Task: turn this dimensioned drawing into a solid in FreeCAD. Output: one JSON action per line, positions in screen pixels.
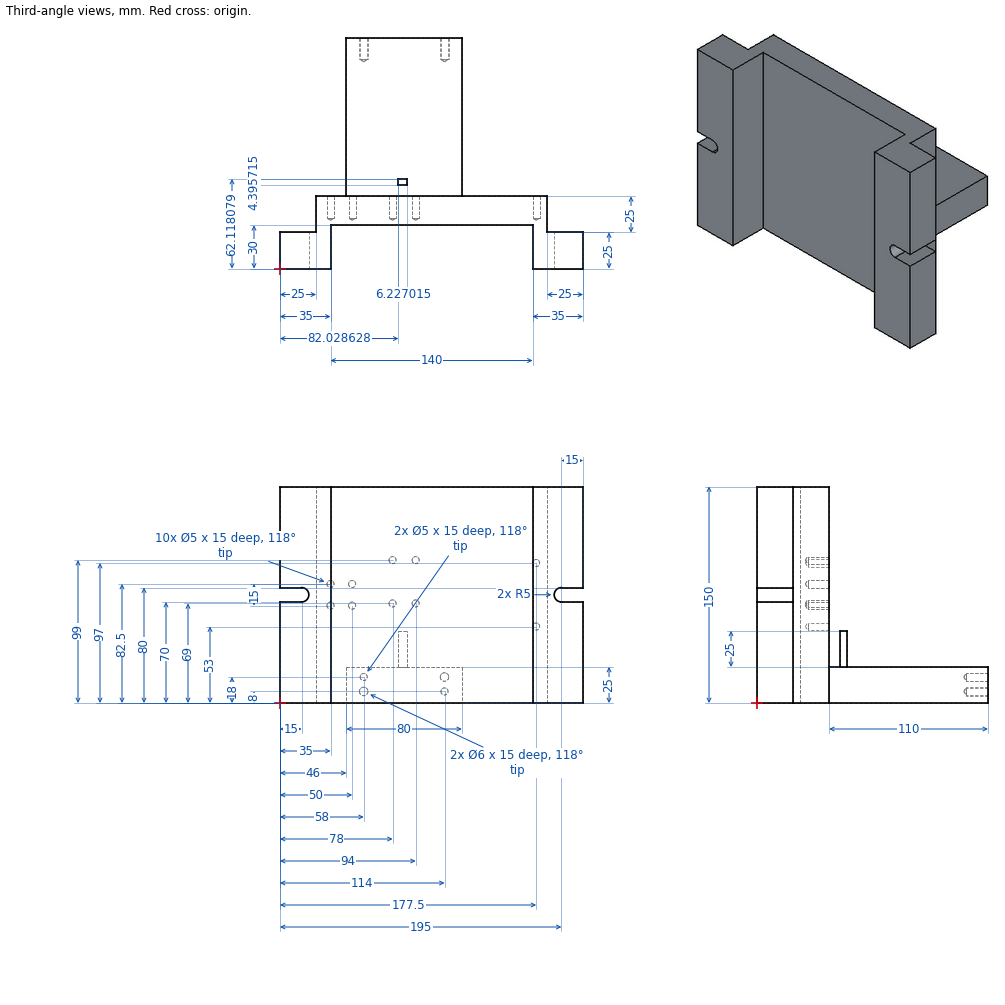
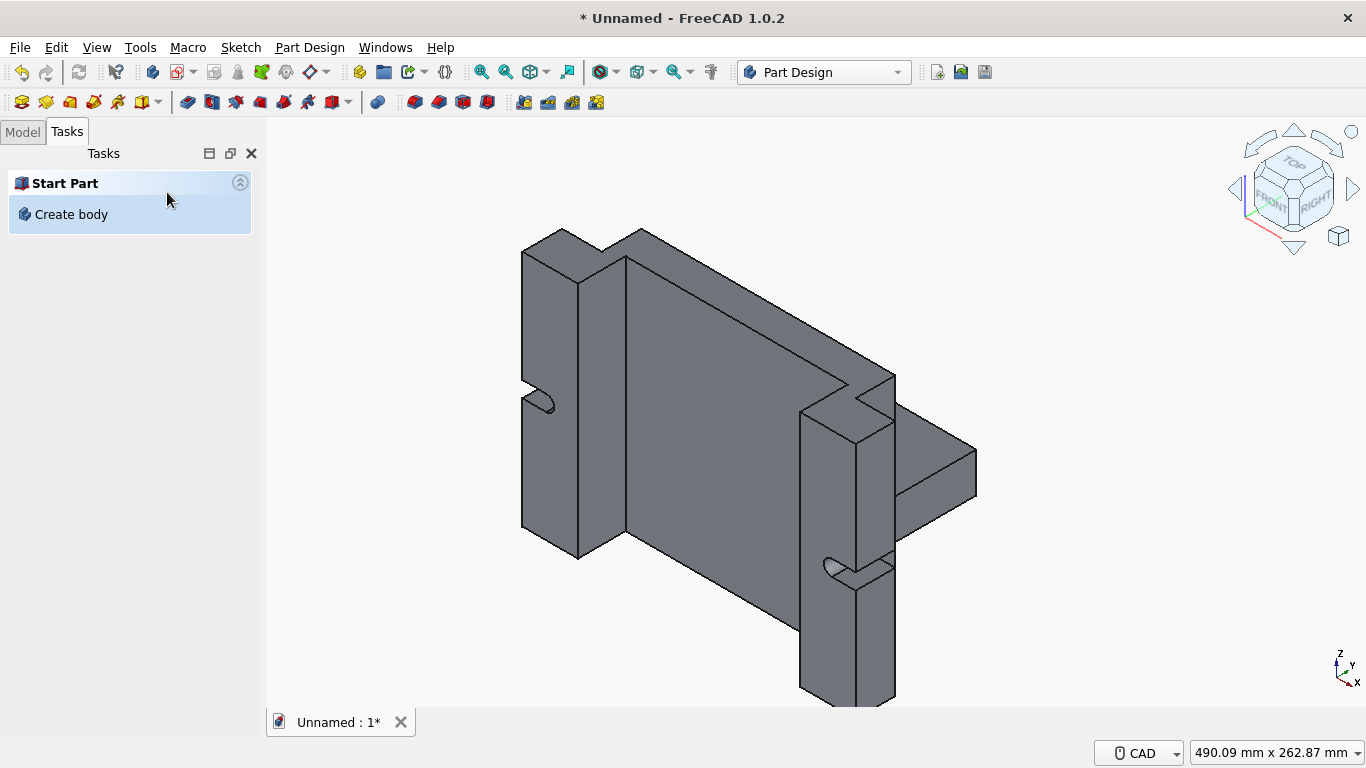
{"action": "left_click", "coordinate": [482, 72]}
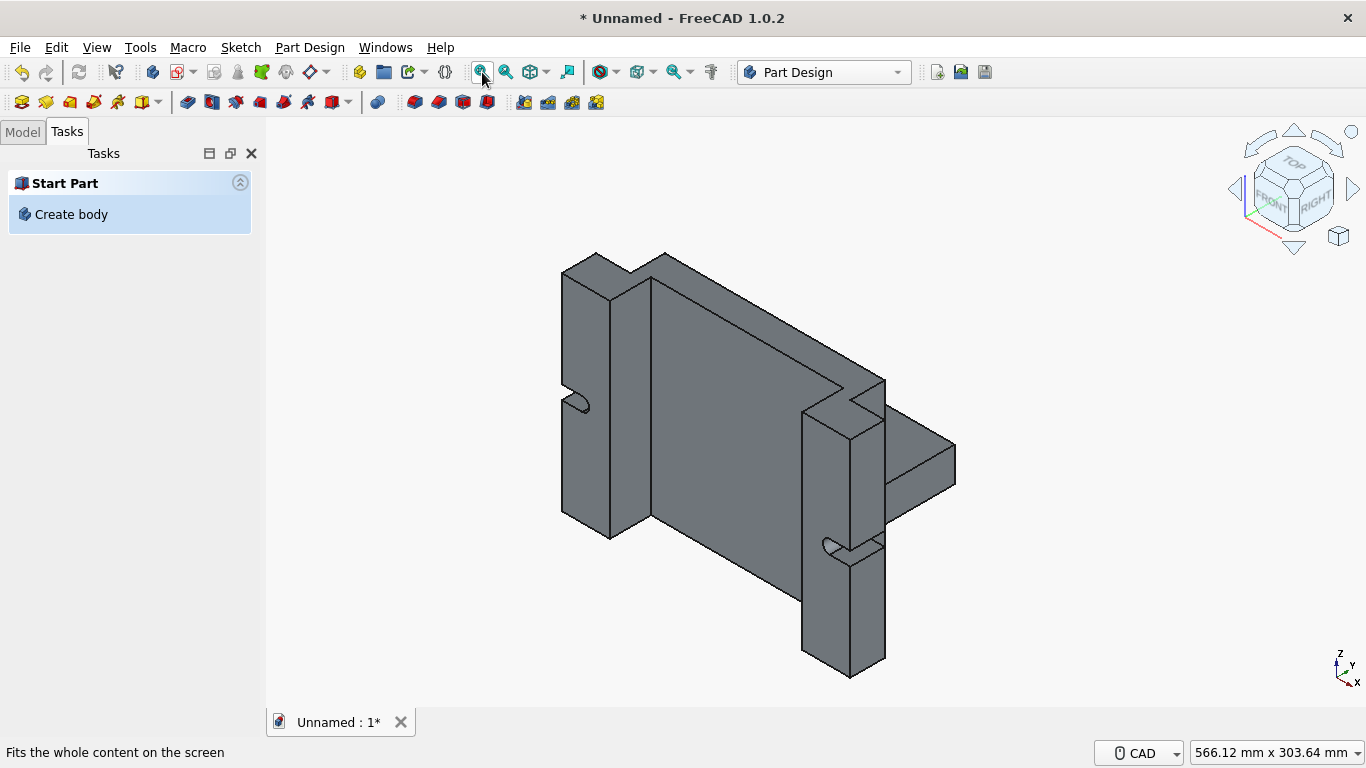
{"action": "key", "text": "2"}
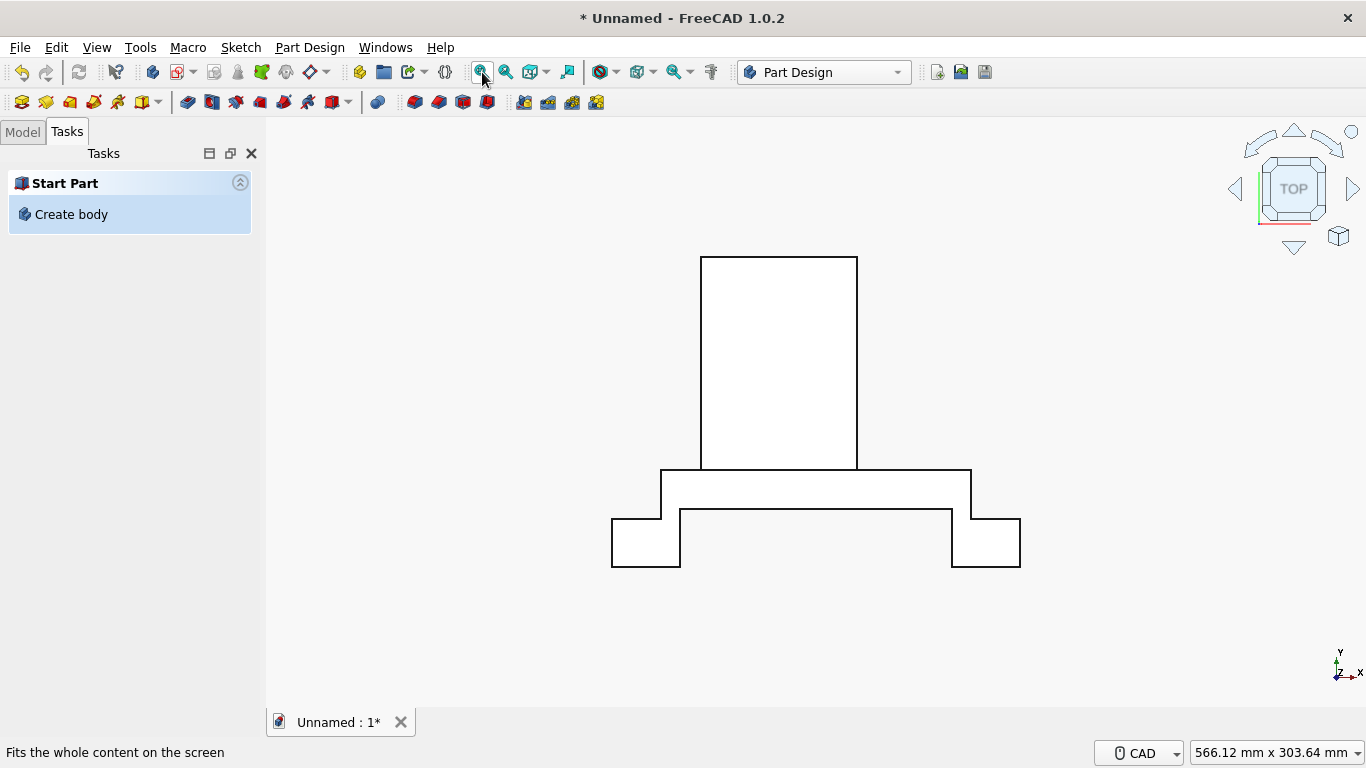
{"action": "left_click", "coordinate": [779, 362]}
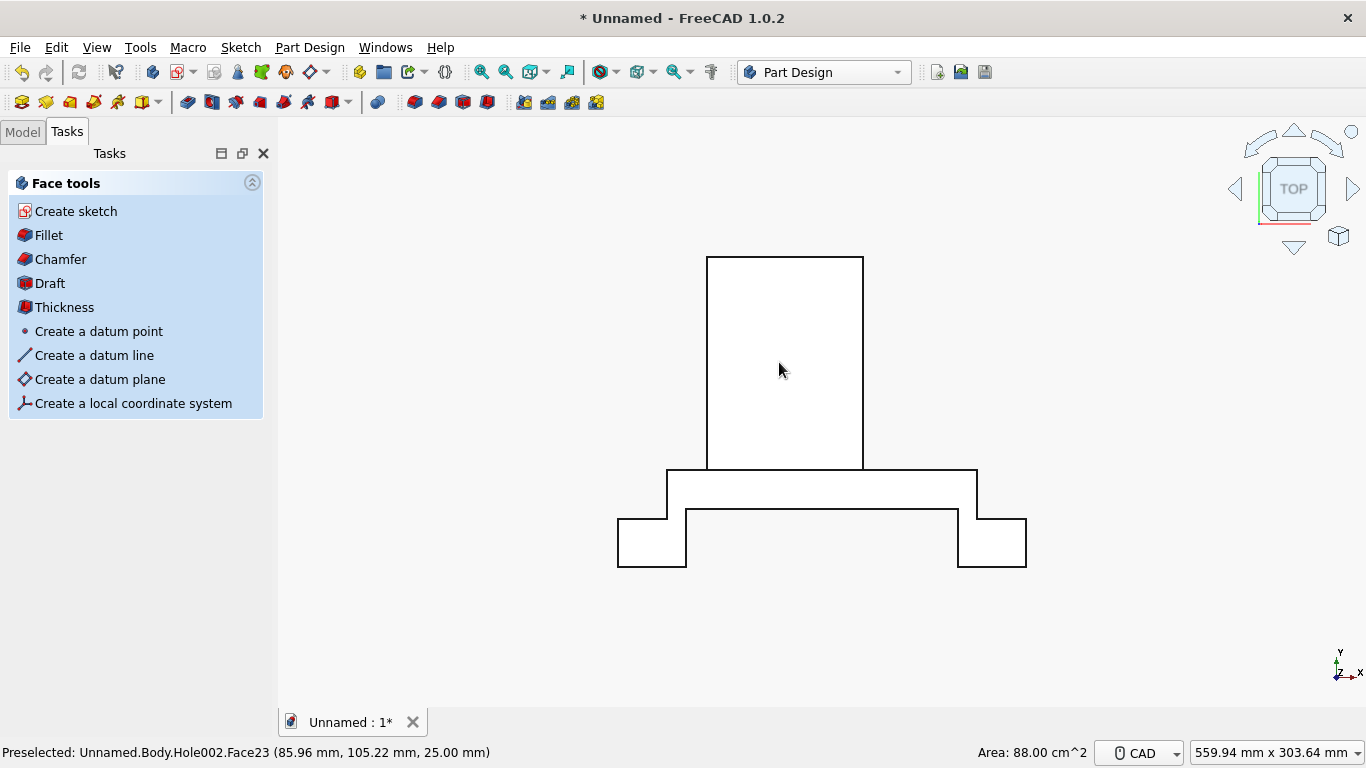
{"action": "left_click", "coordinate": [178, 72]}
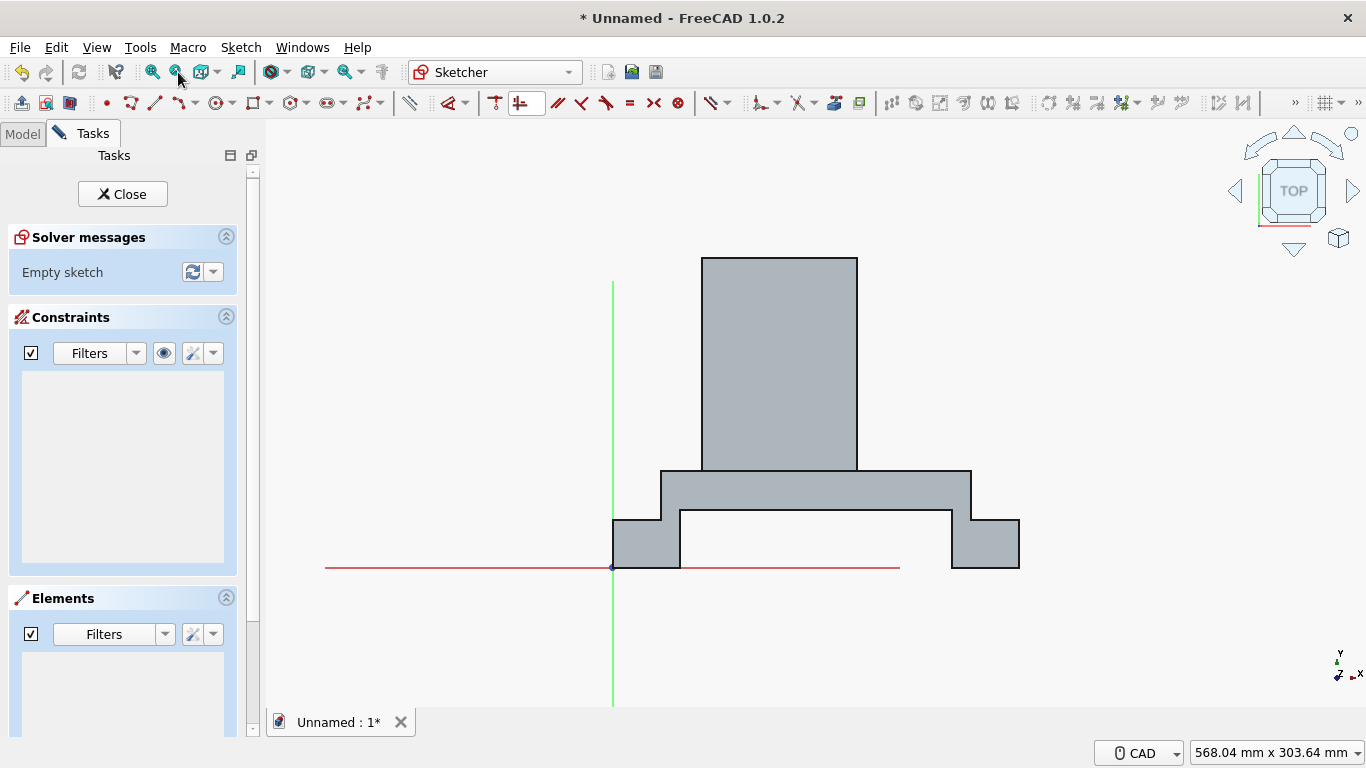
{"action": "left_click", "coordinate": [70, 104]}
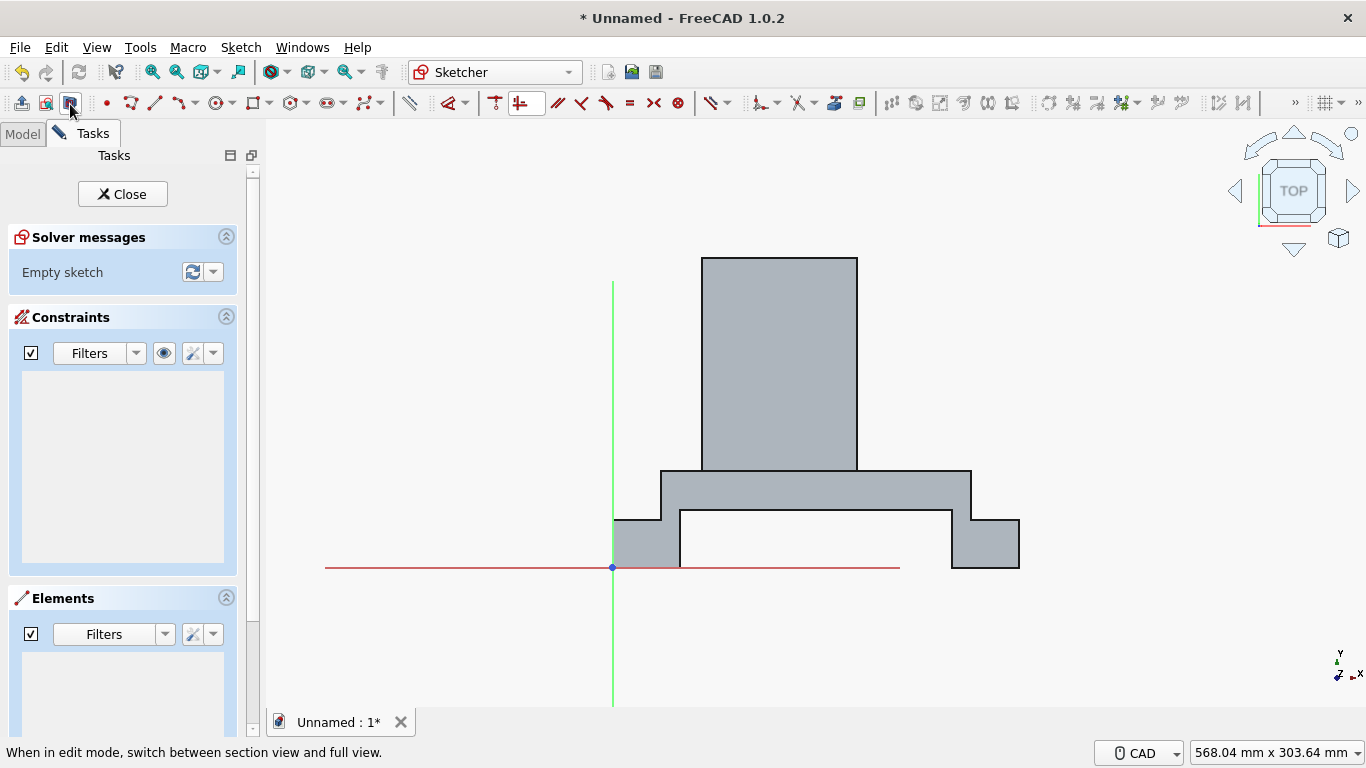
{"action": "scroll", "coordinate": [779, 454], "scroll_direction": "up", "scroll_amount": 15}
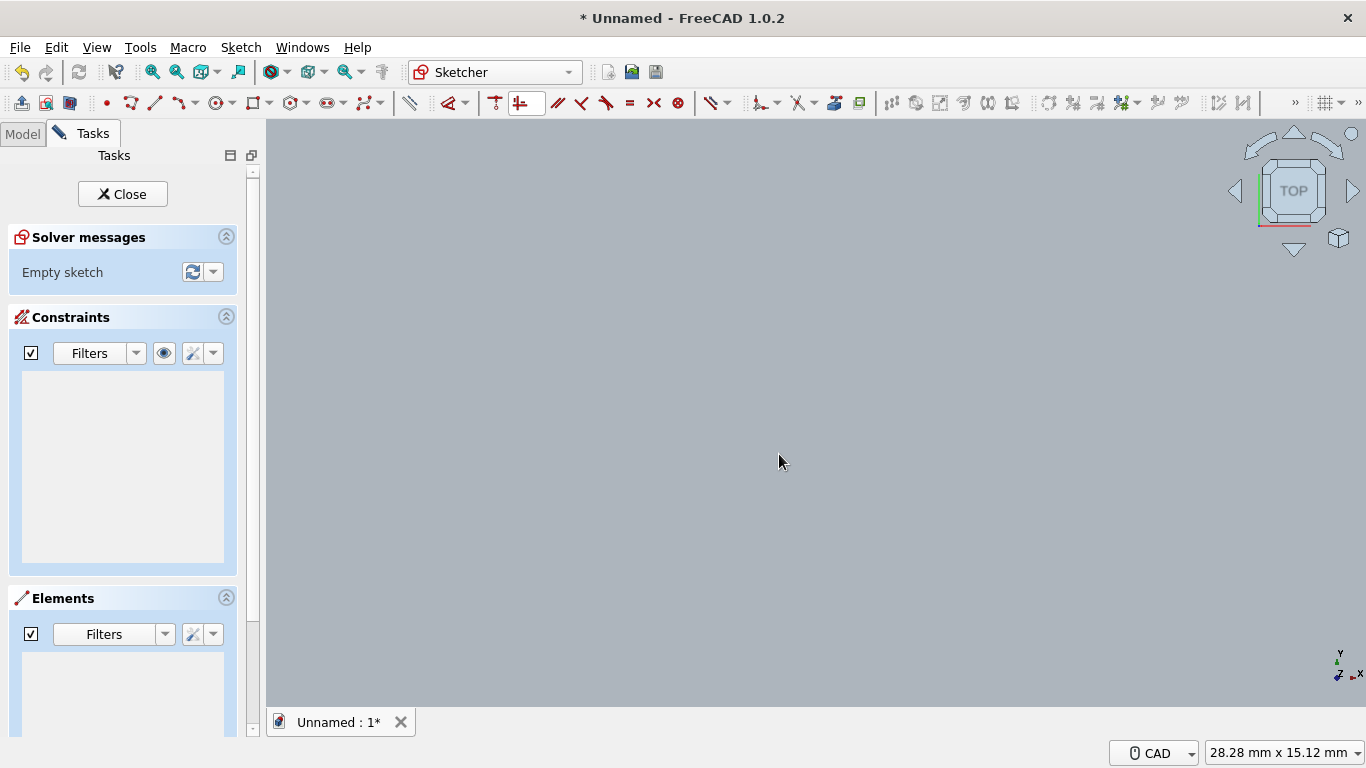
{"action": "scroll", "coordinate": [735, 390], "scroll_direction": "up", "scroll_amount": 4}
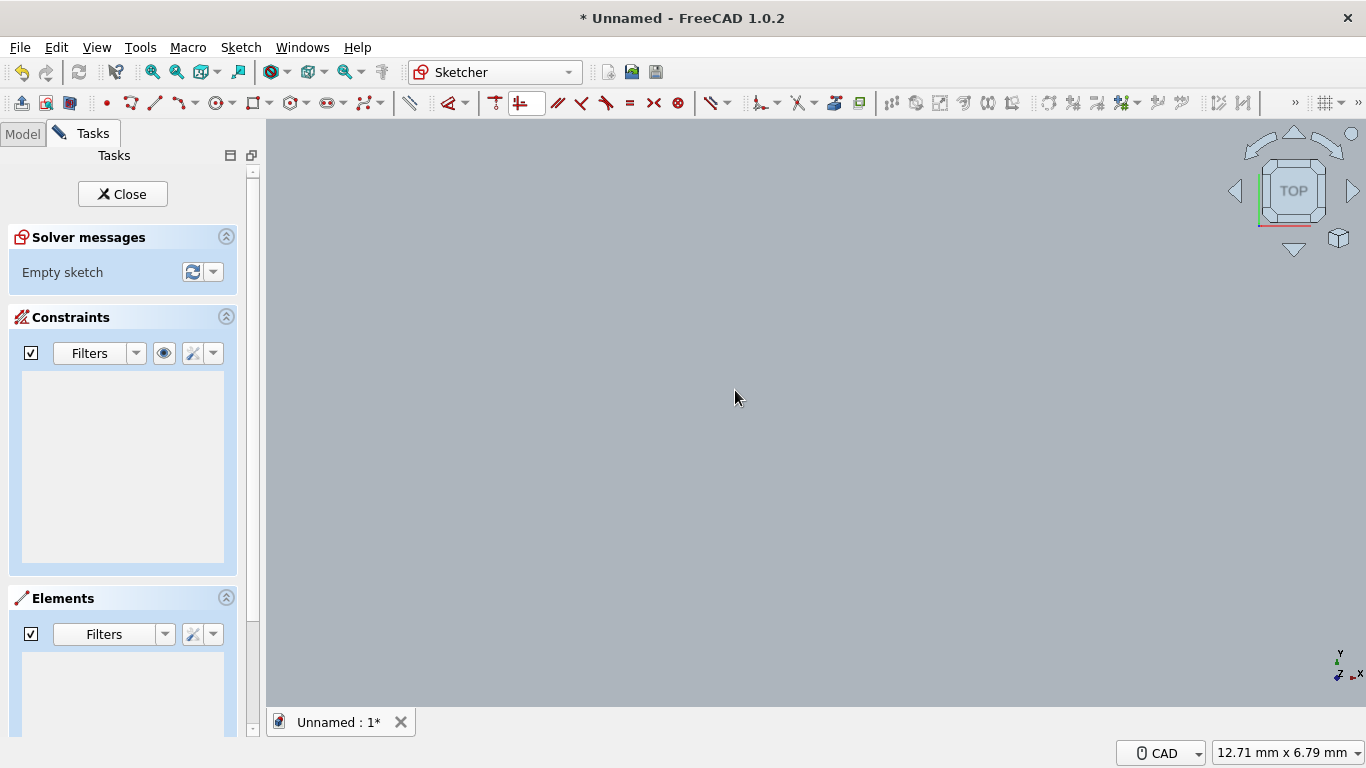
{"action": "key", "text": "g r"}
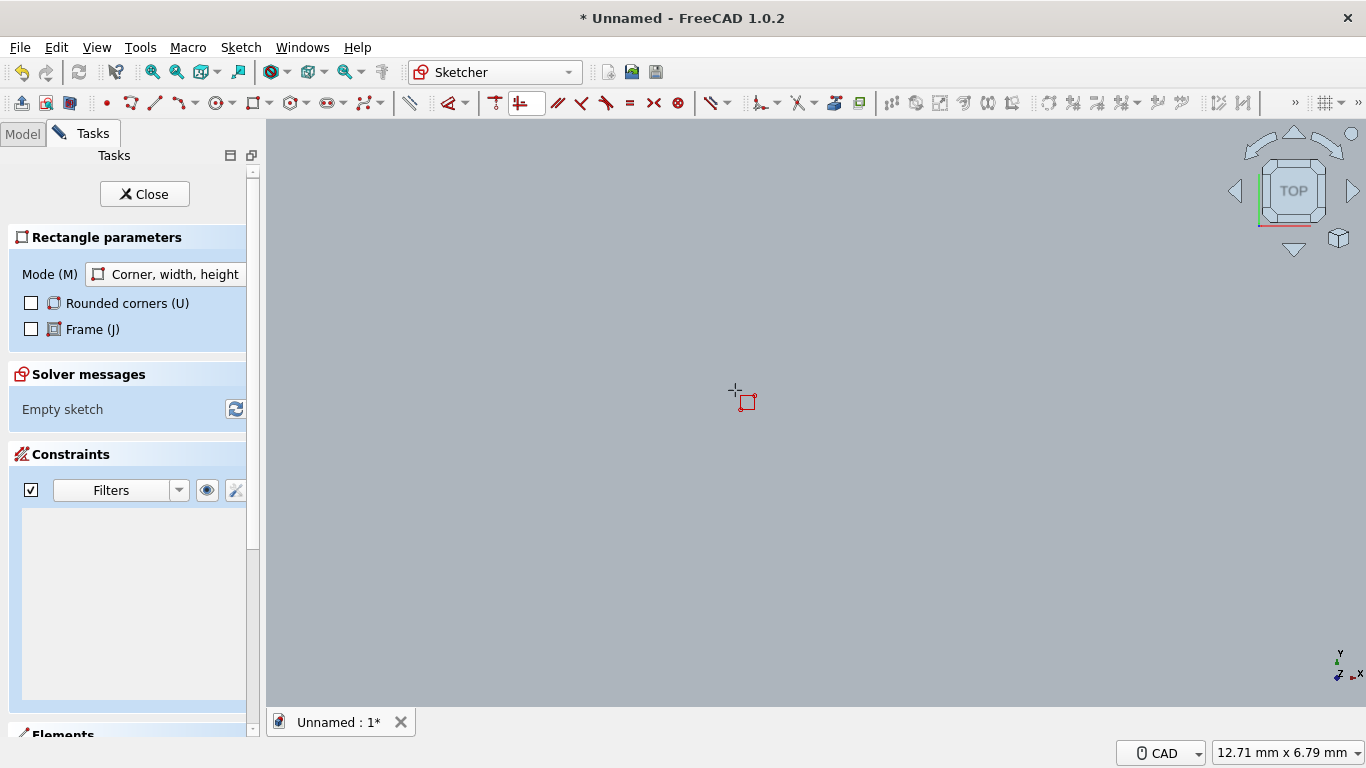
{"action": "left_click", "coordinate": [478, 223]}
{"action": "mouse_move", "coordinate": [1017, 603]}